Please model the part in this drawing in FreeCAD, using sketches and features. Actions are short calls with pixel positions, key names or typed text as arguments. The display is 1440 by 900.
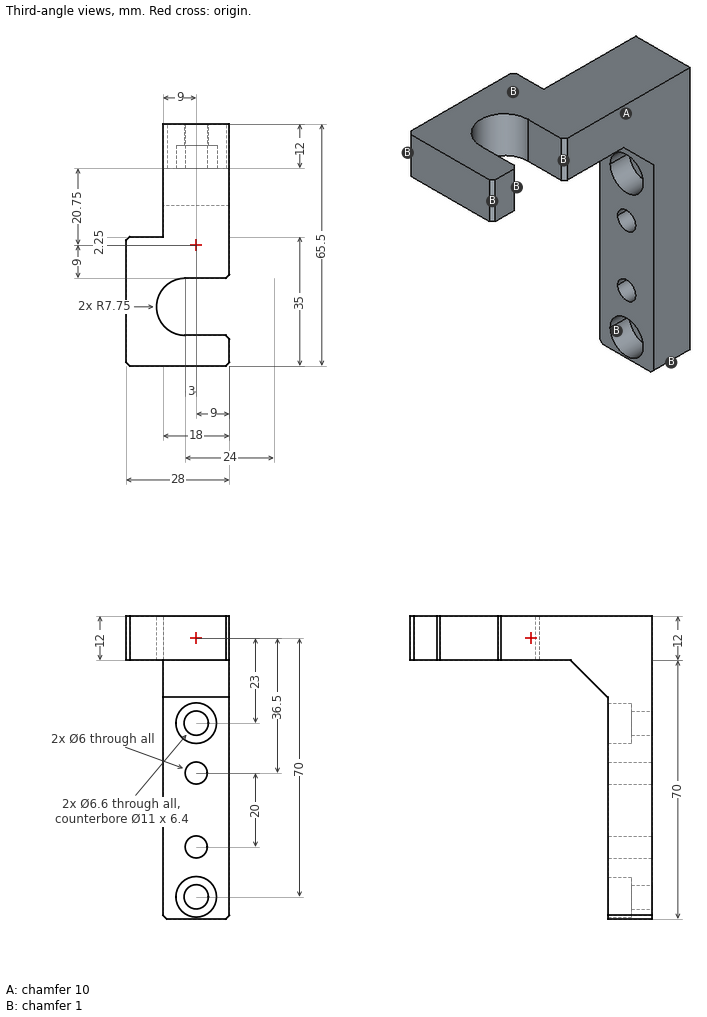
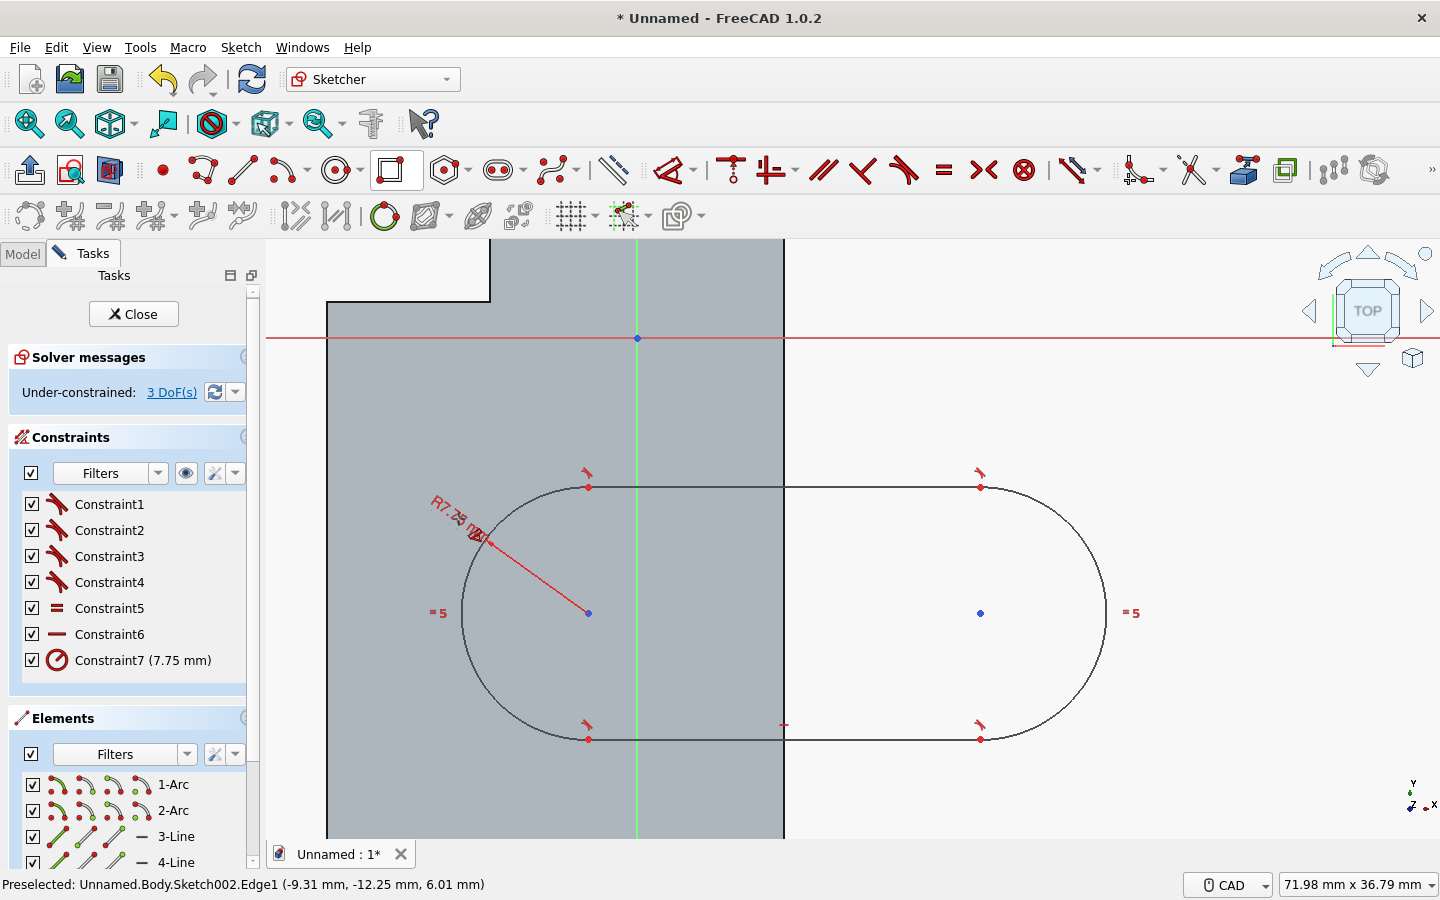
click(706, 487)
click(784, 453)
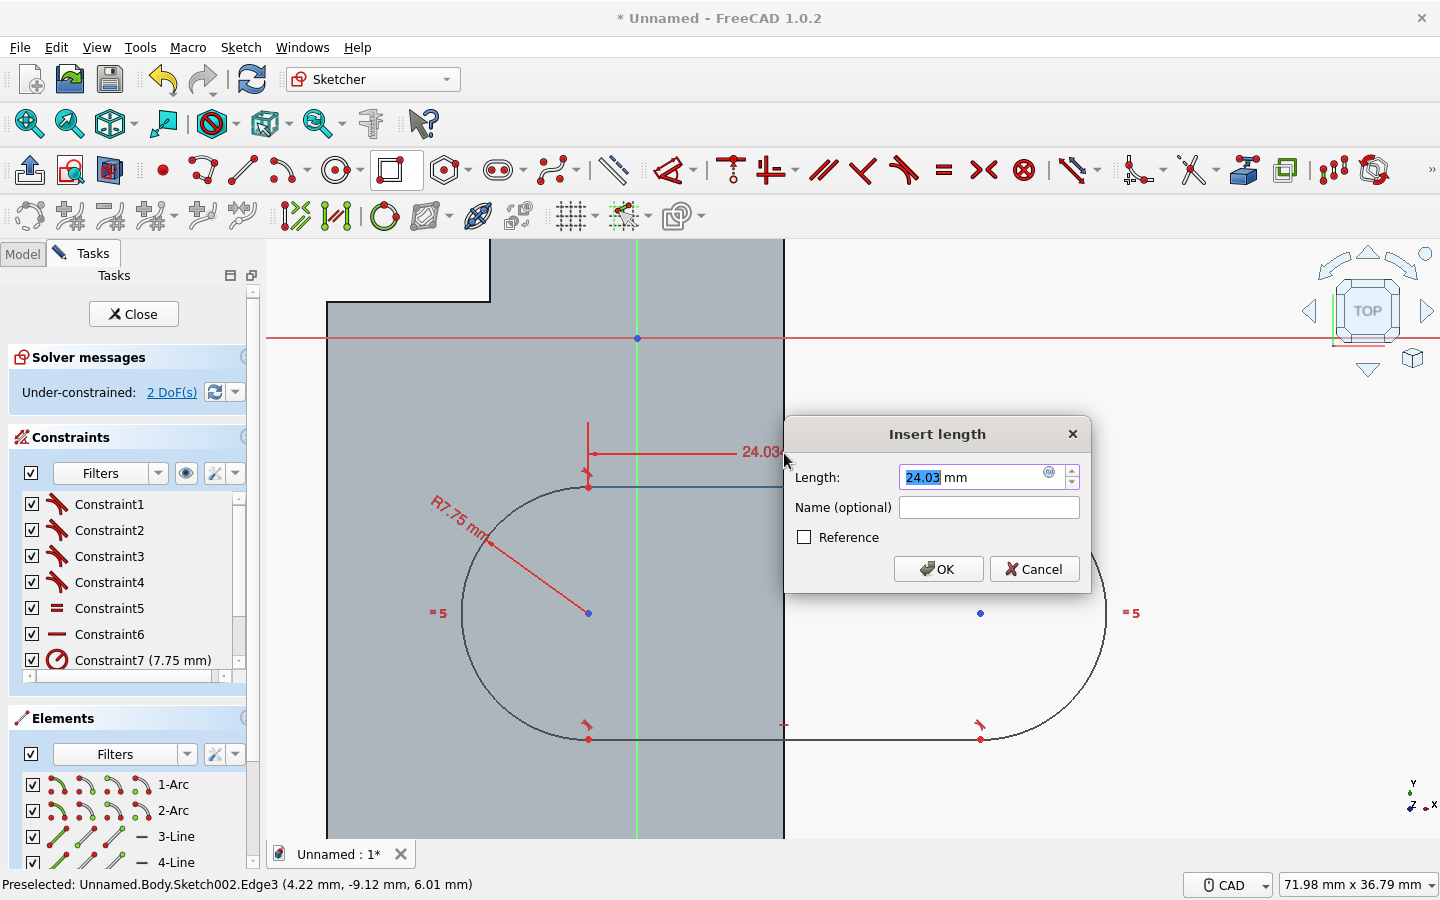
text(24)
key(Return)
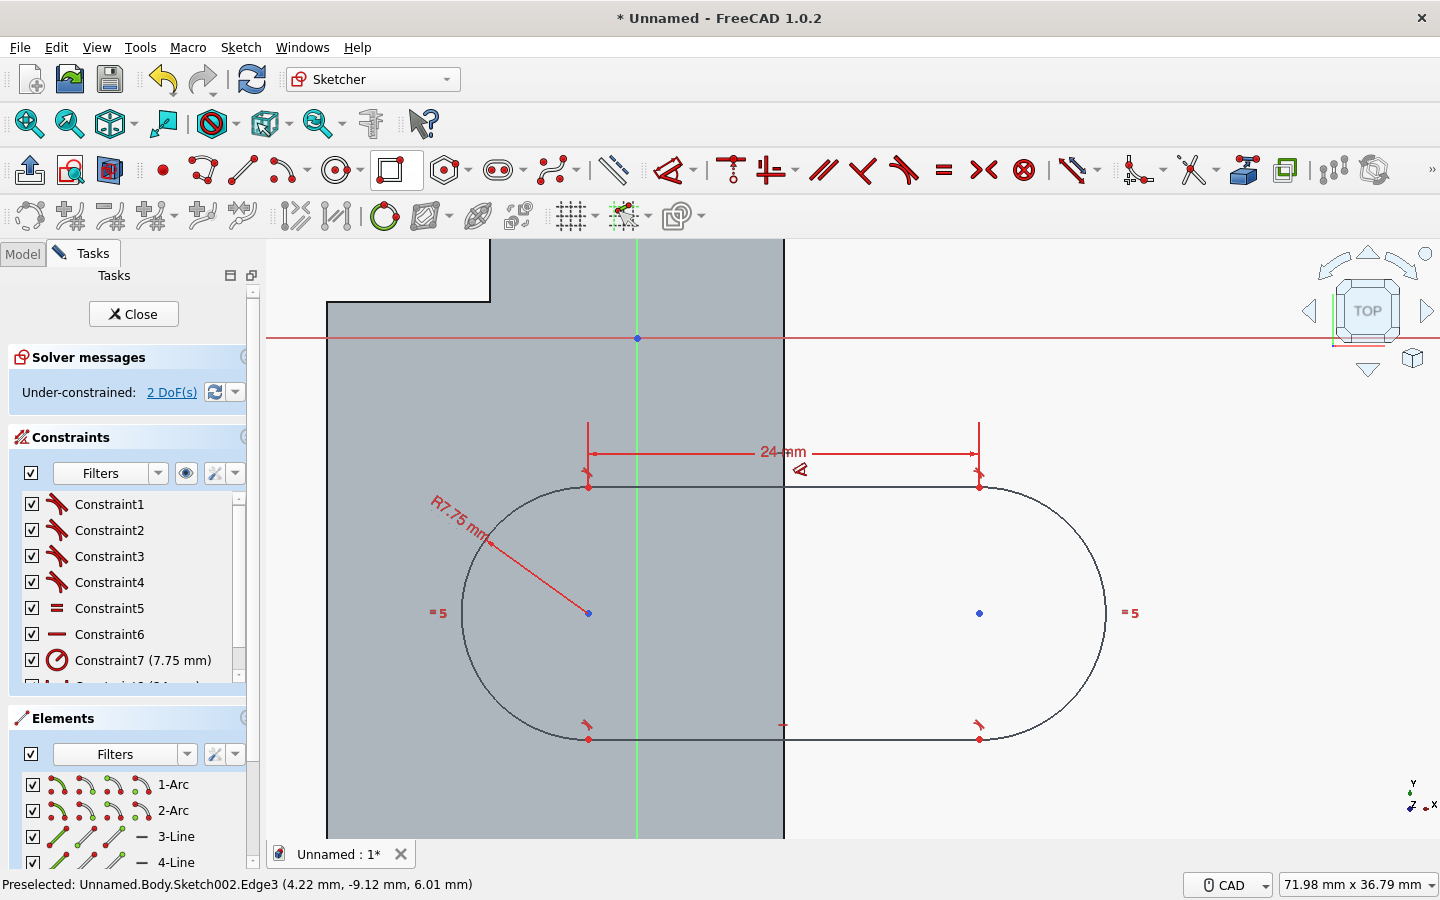
click(588, 487)
click(613, 304)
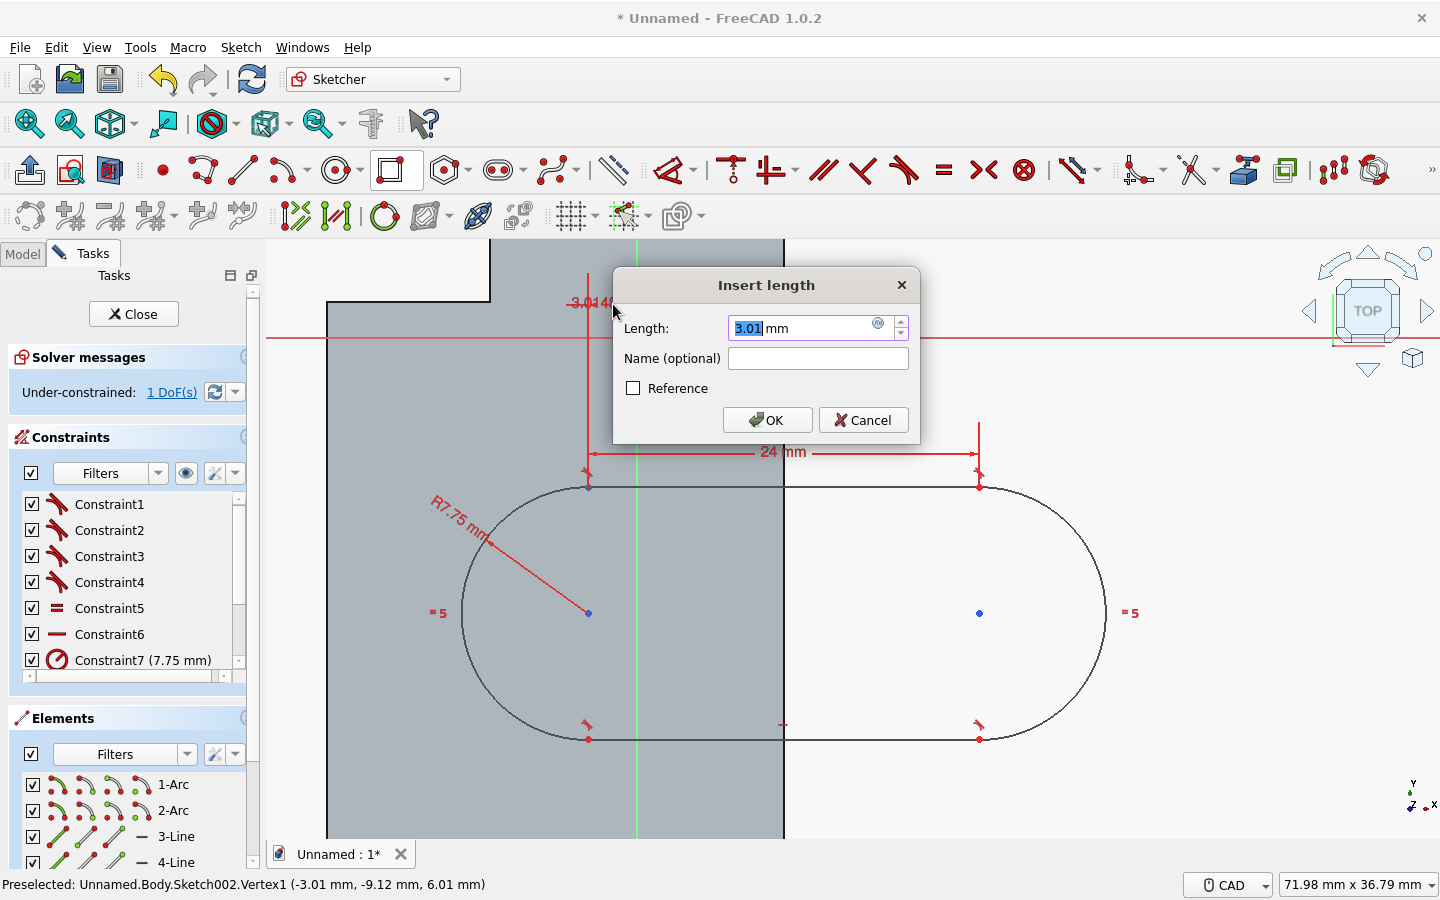
text(3)
key(Return)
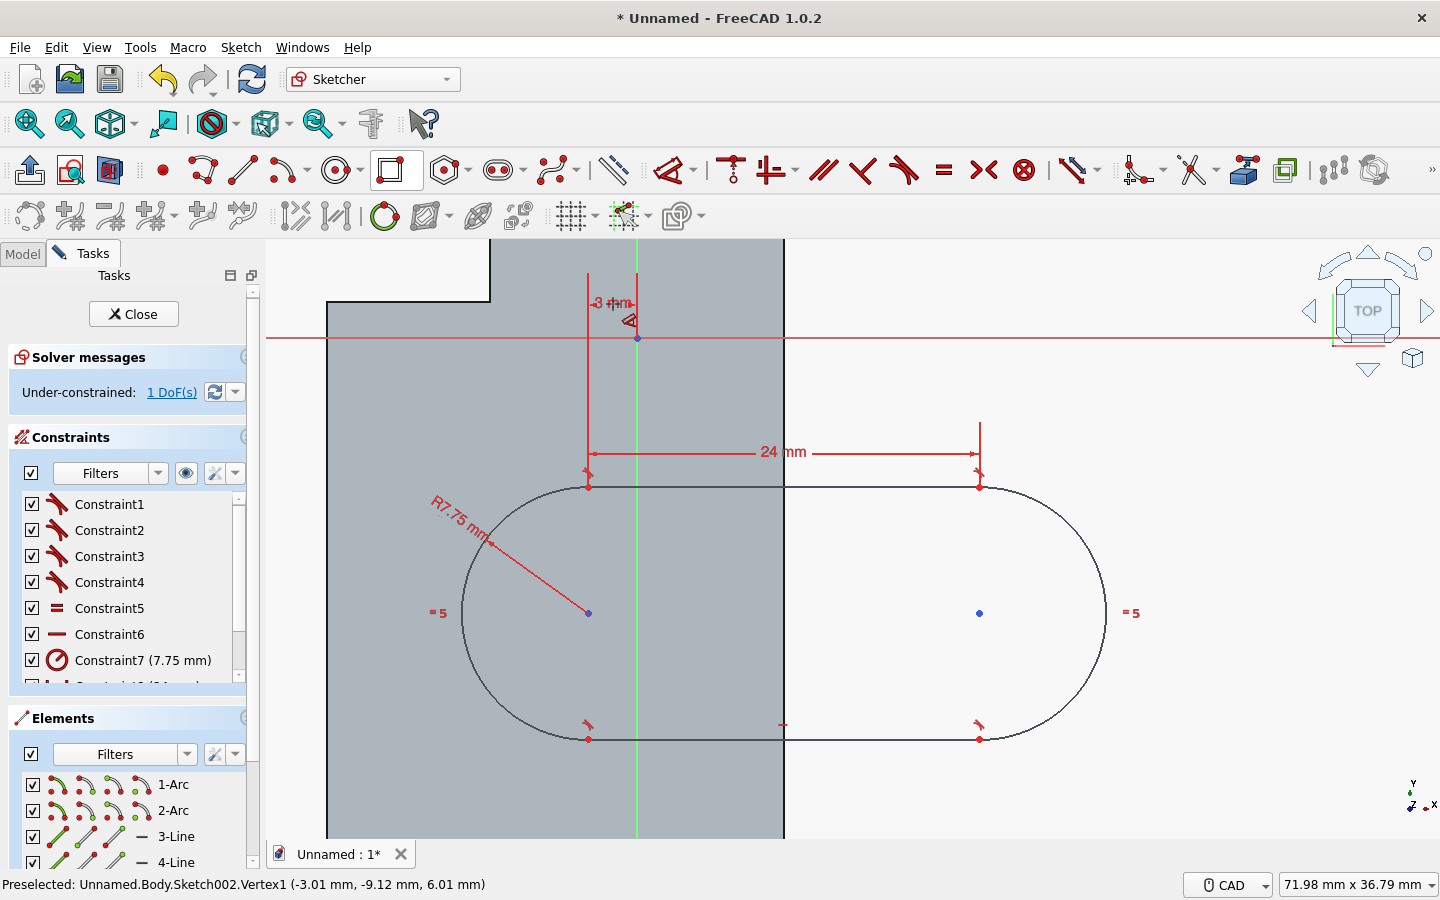
click(588, 487)
click(554, 413)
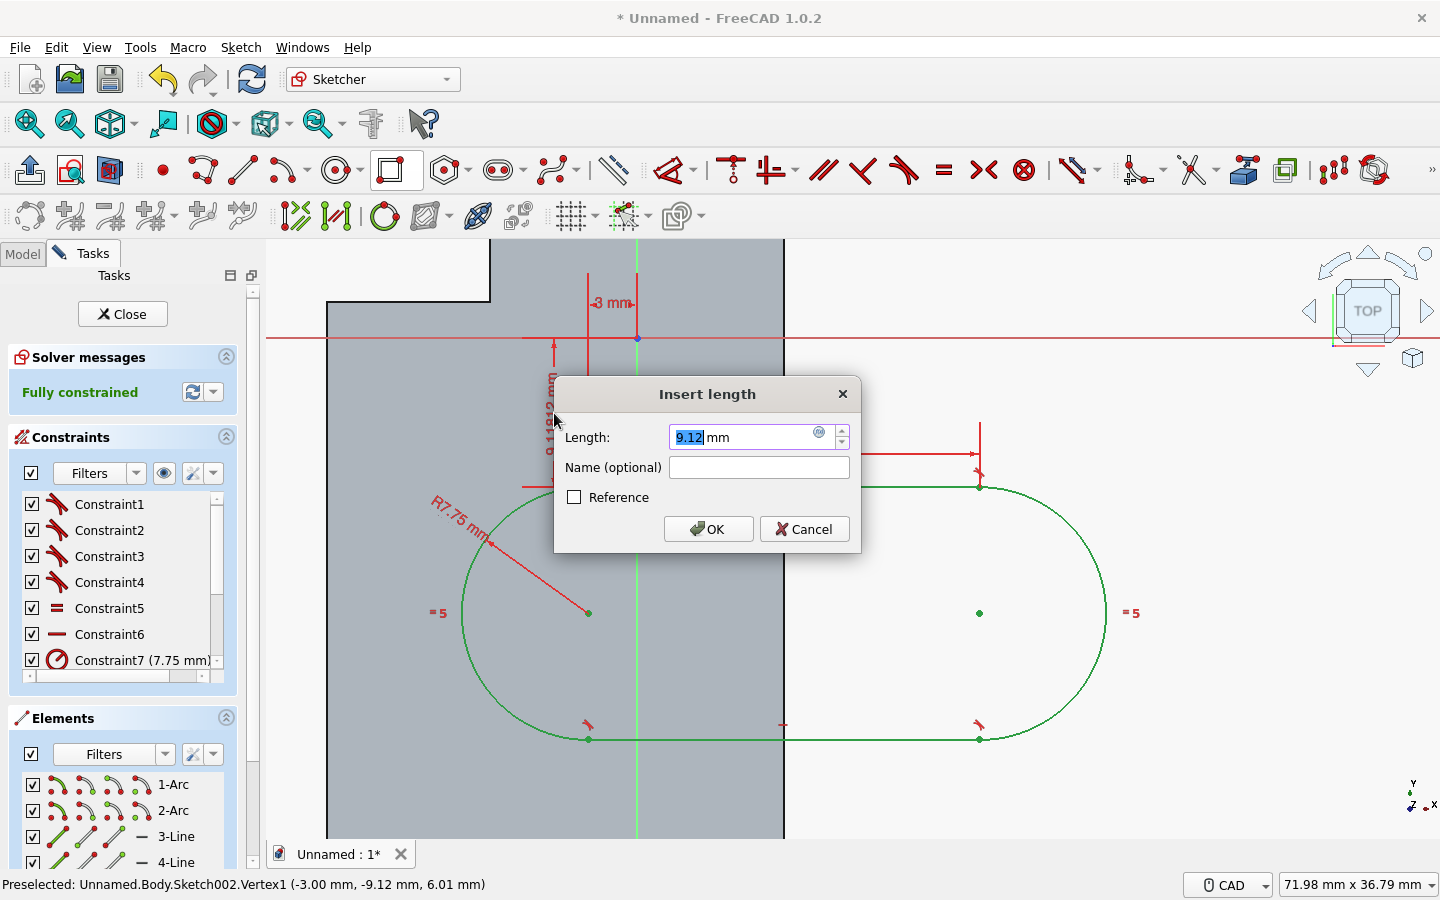
text(9)
key(Return)
key(Escape)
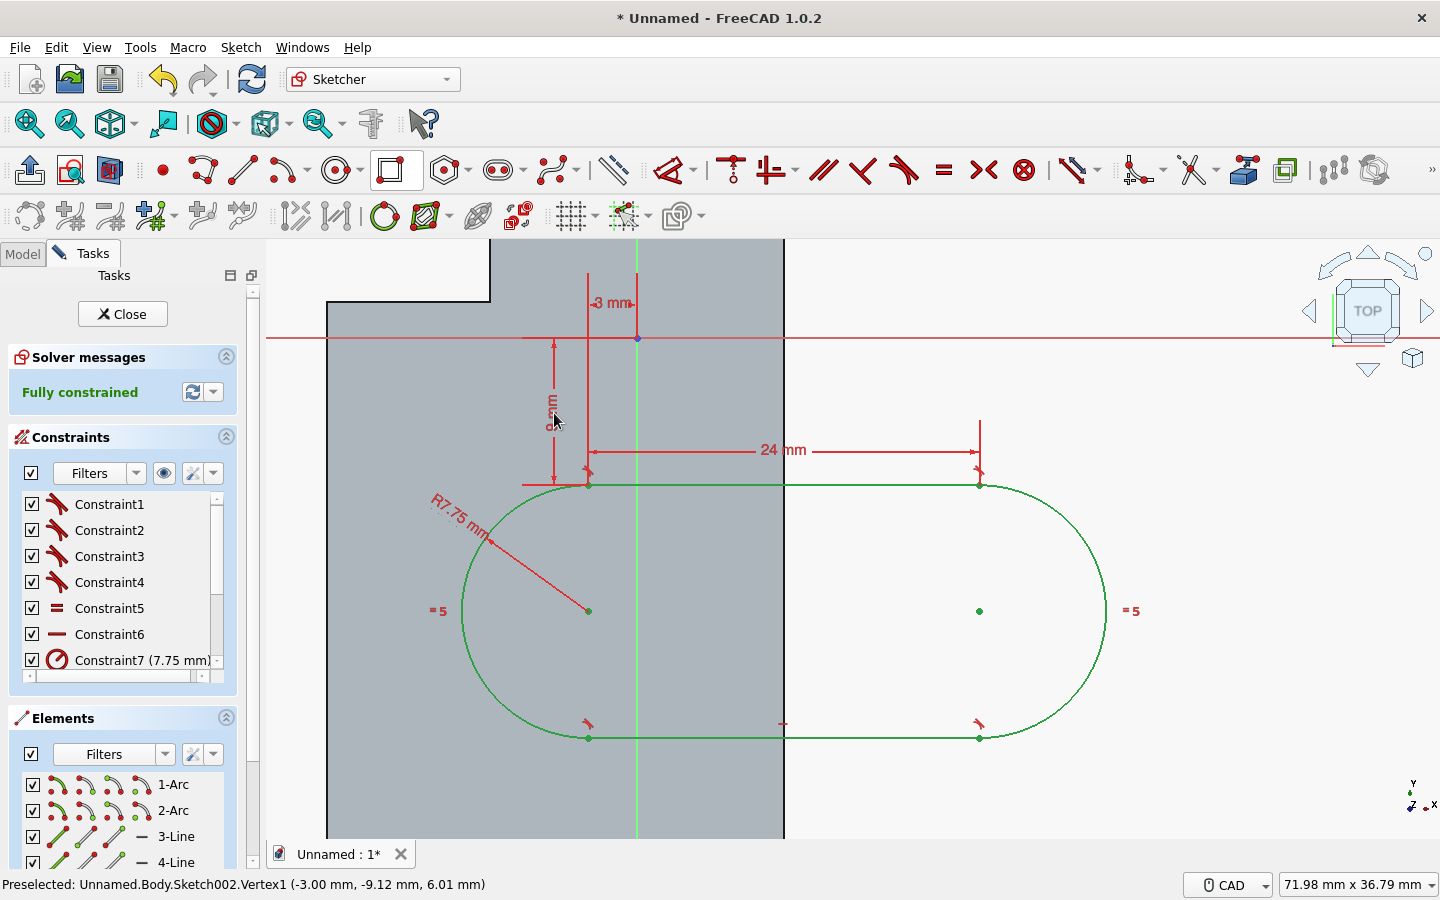
click(123, 314)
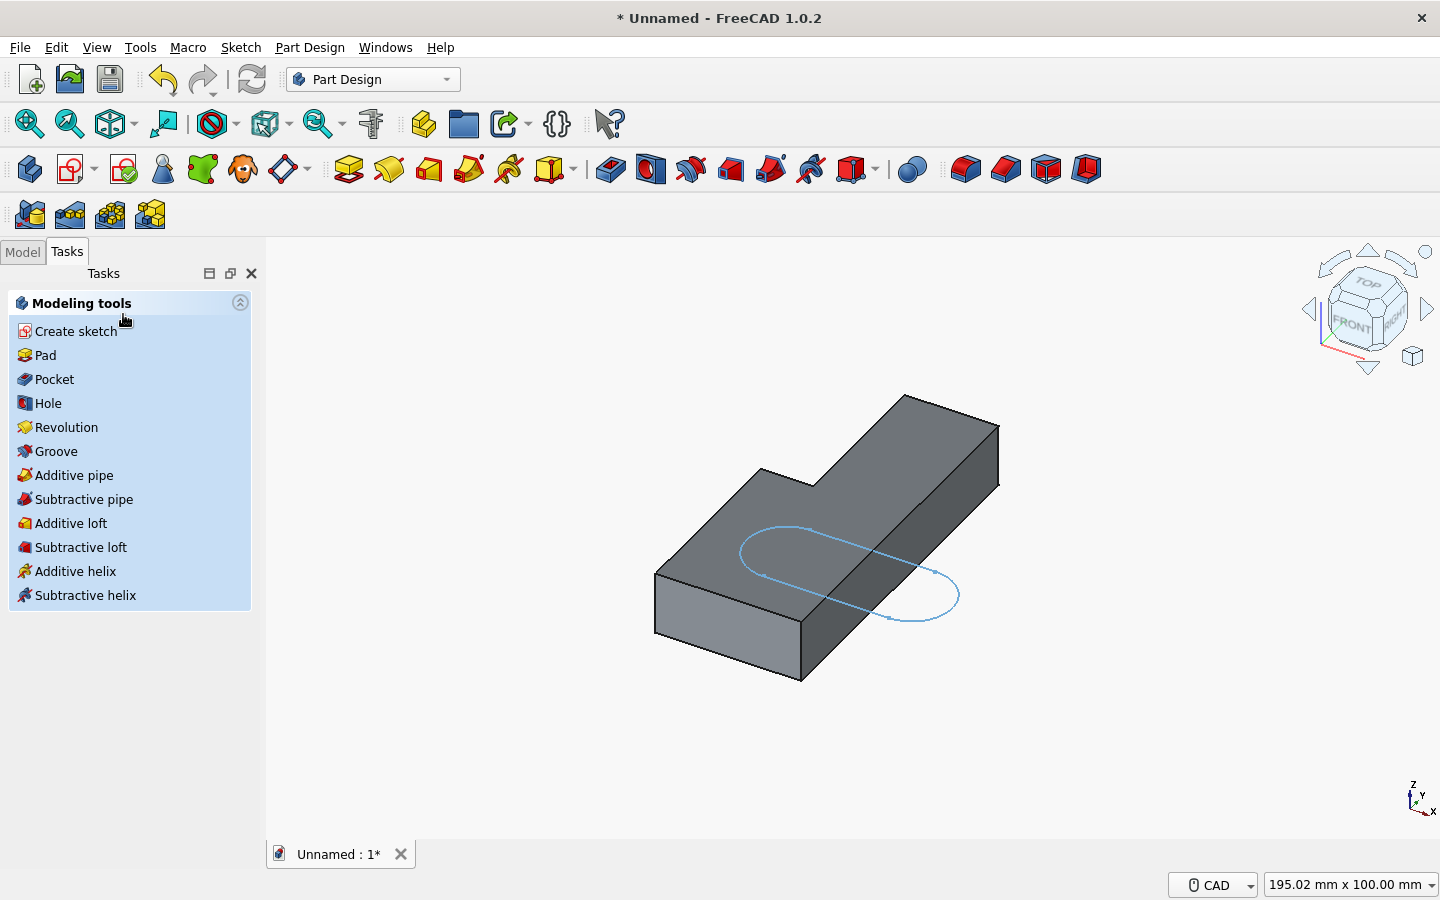
click(612, 170)